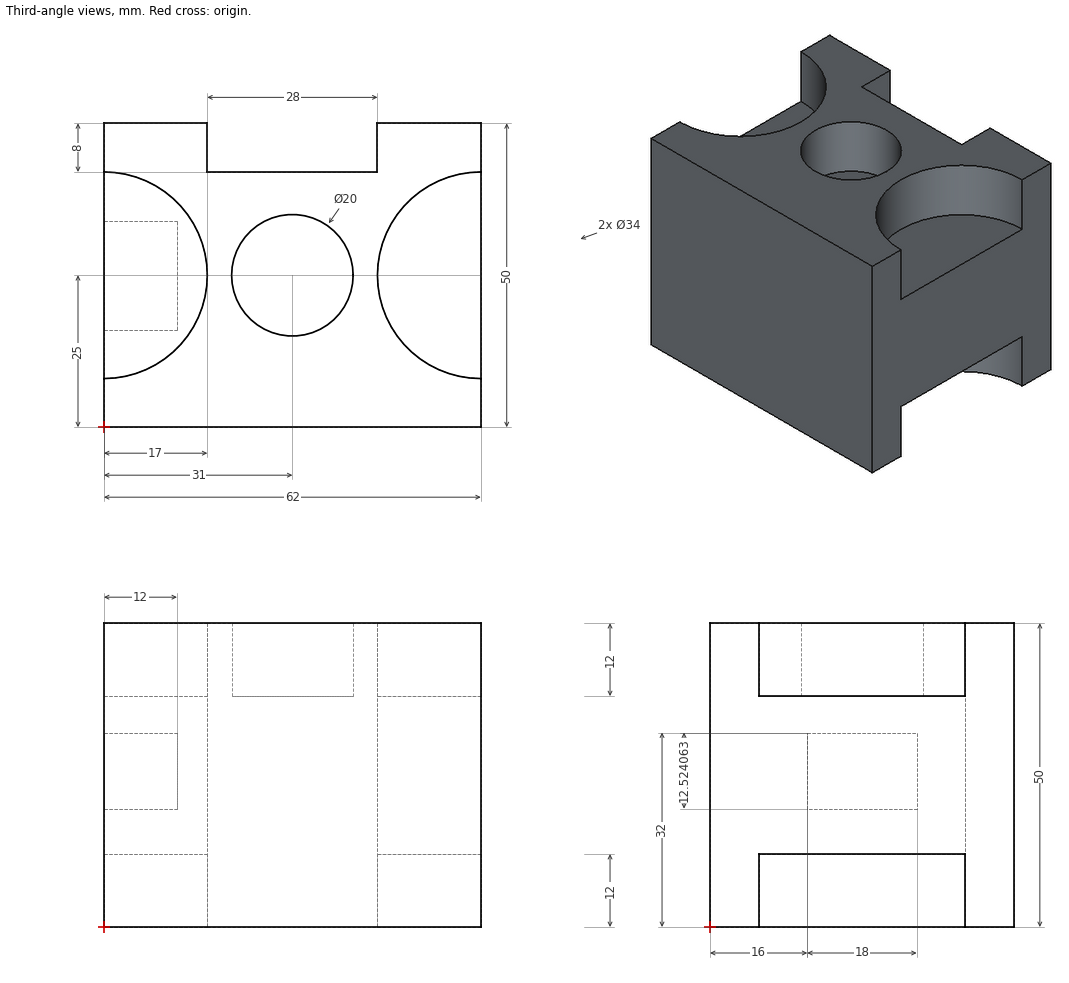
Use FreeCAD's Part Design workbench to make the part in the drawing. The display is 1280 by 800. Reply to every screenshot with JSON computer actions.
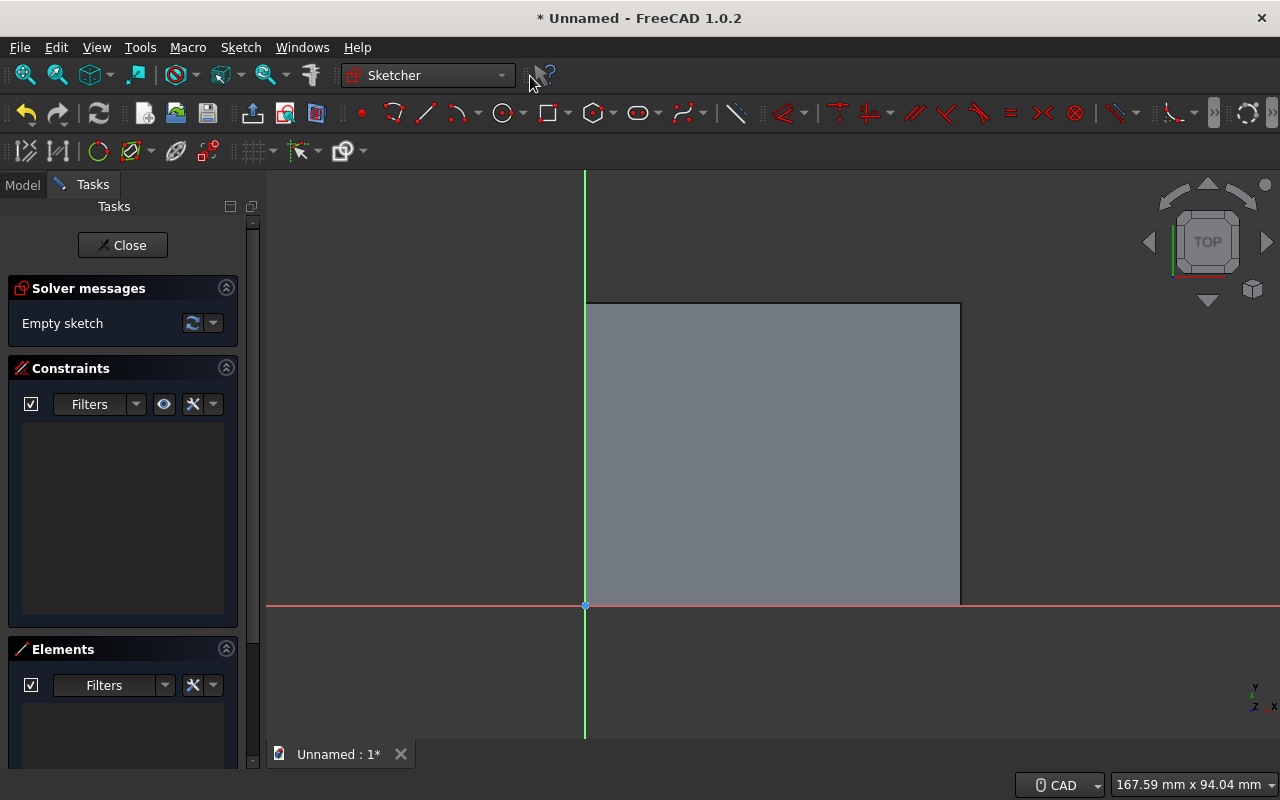
{"action": "left_click", "coordinate": [504, 114]}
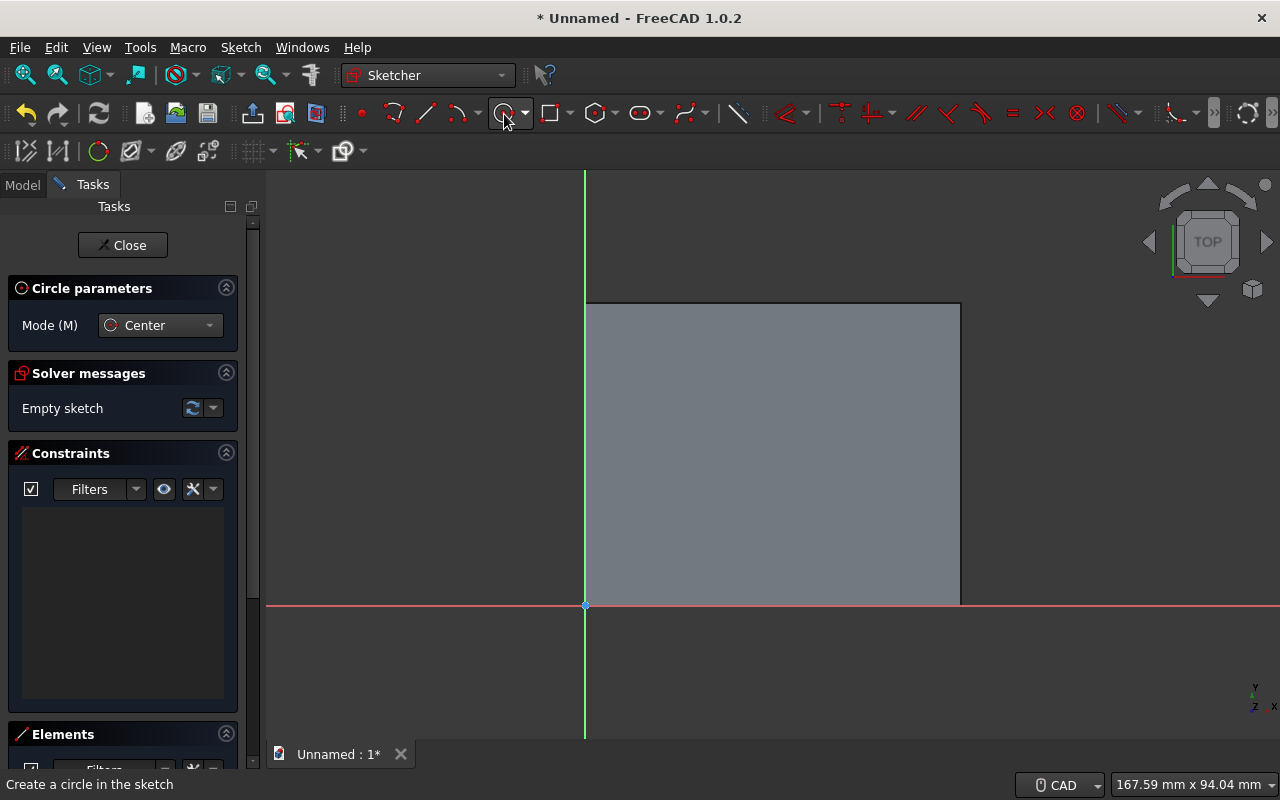
{"action": "left_click", "coordinate": [961, 455]}
{"action": "left_click", "coordinate": [1033, 382]}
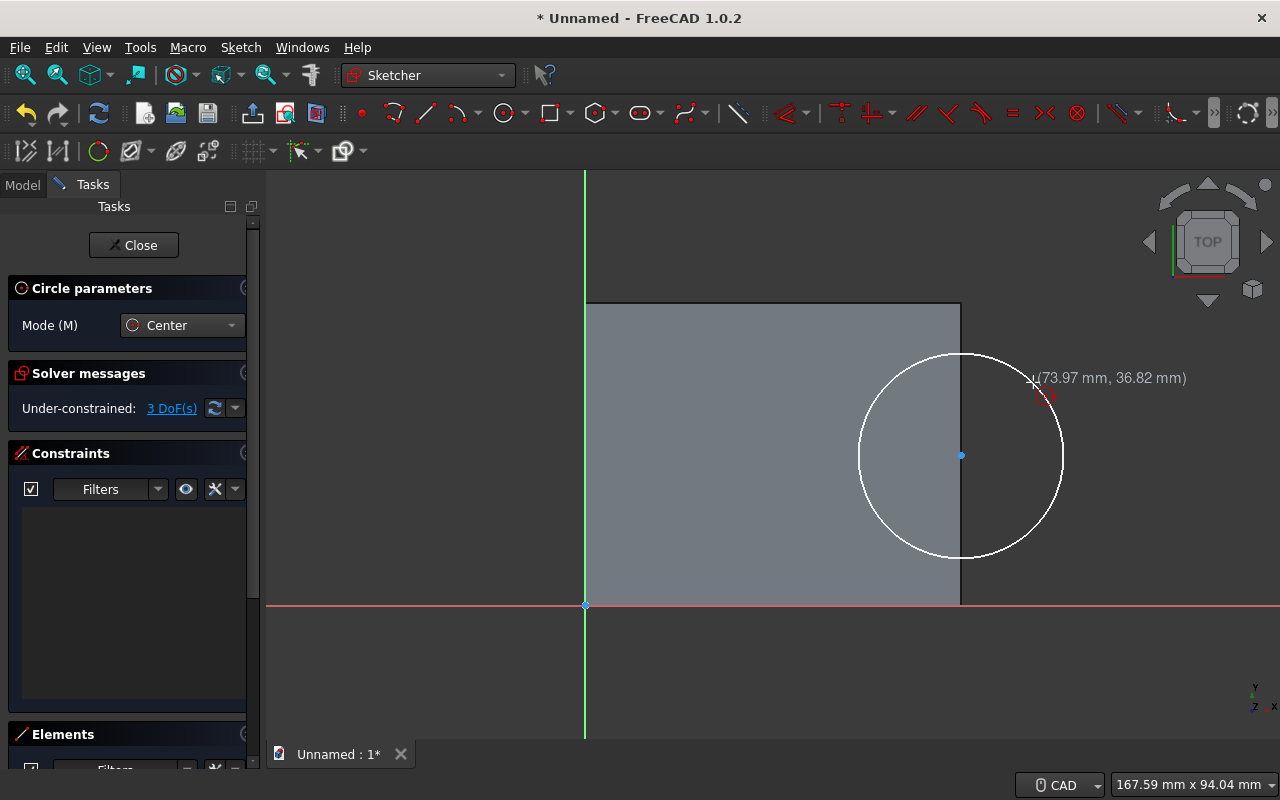
{"action": "left_click", "coordinate": [585, 455]}
{"action": "left_click", "coordinate": [658, 382]}
{"action": "key", "text": "Escape"}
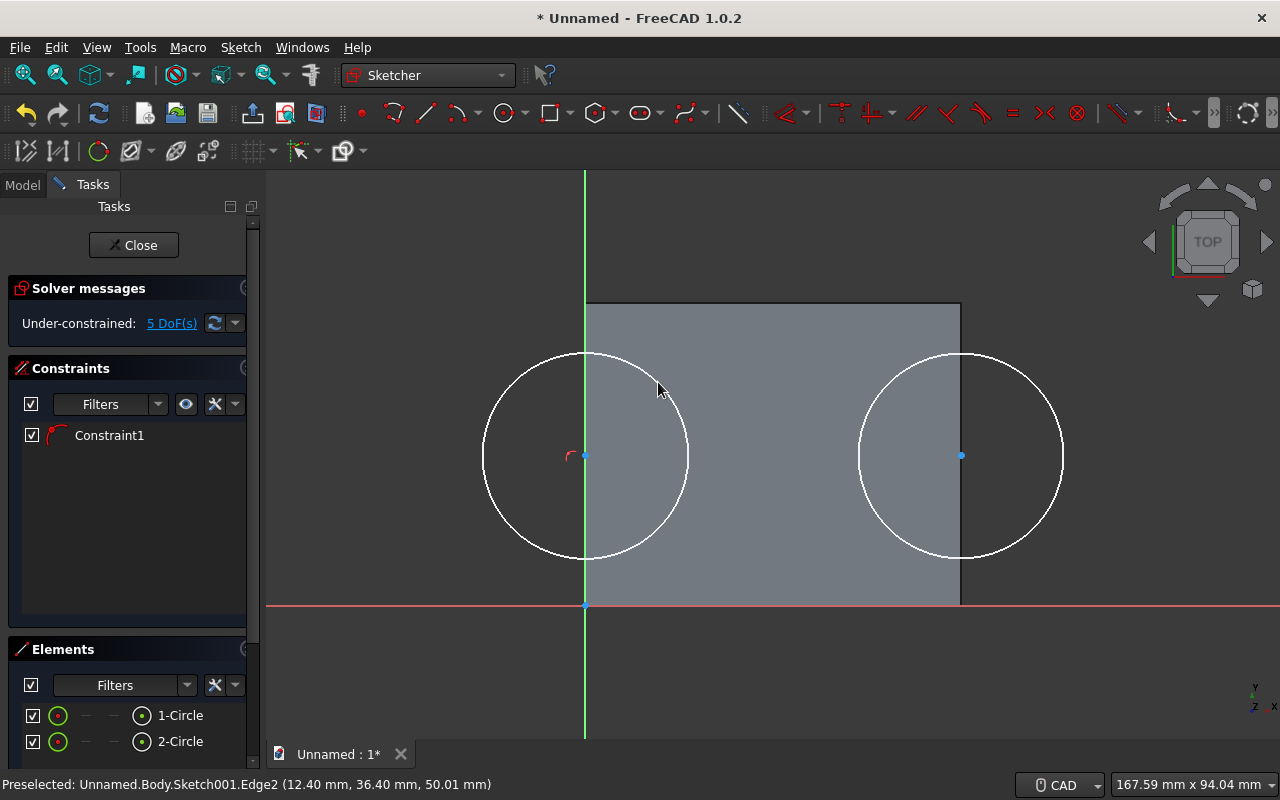
{"action": "left_click", "coordinate": [1033, 383]}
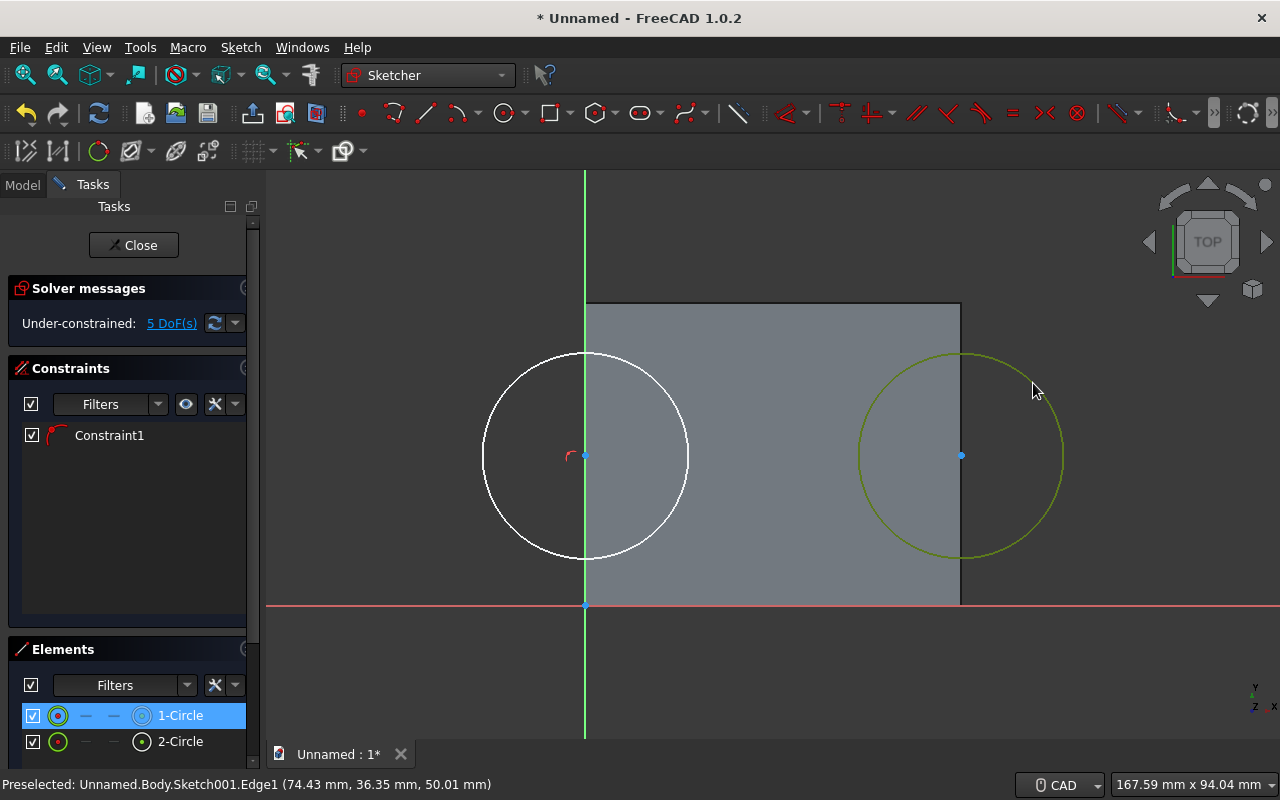
{"action": "left_click", "coordinate": [658, 383]}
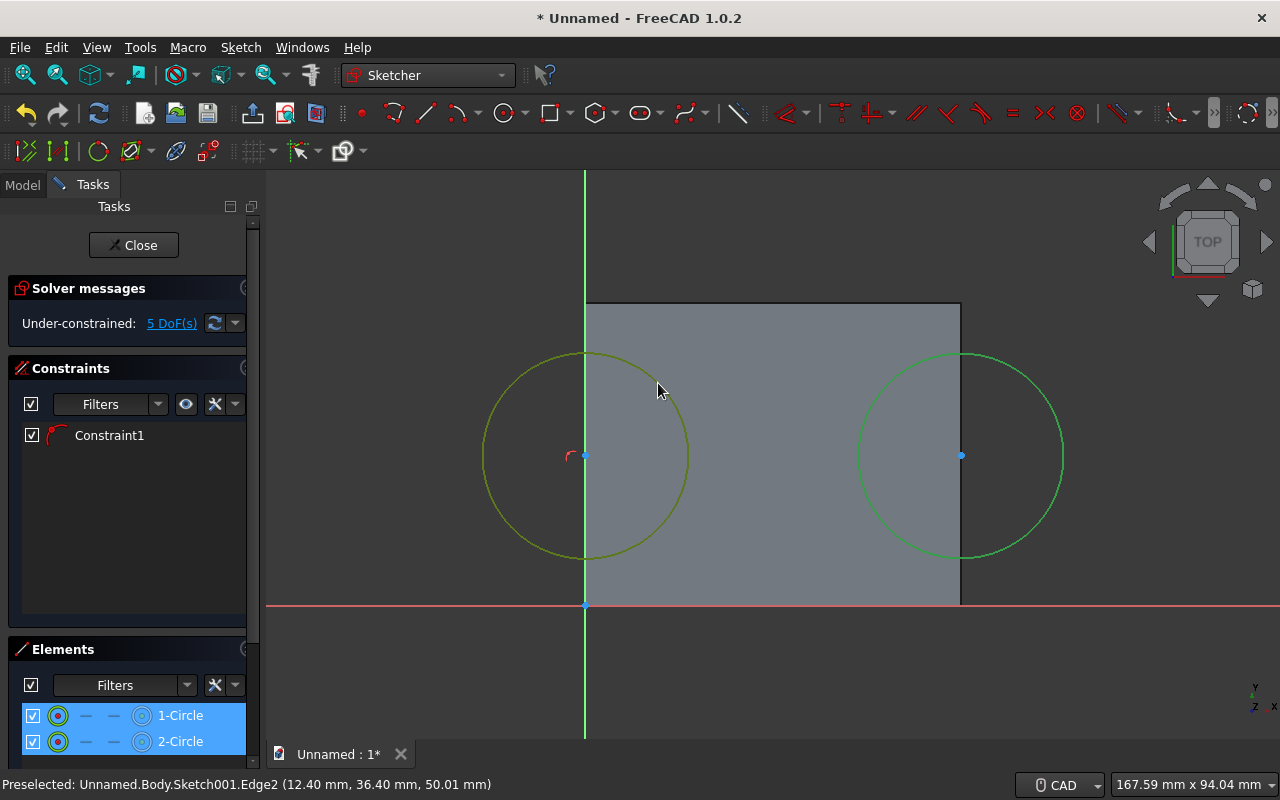
{"action": "left_click", "coordinate": [1014, 114]}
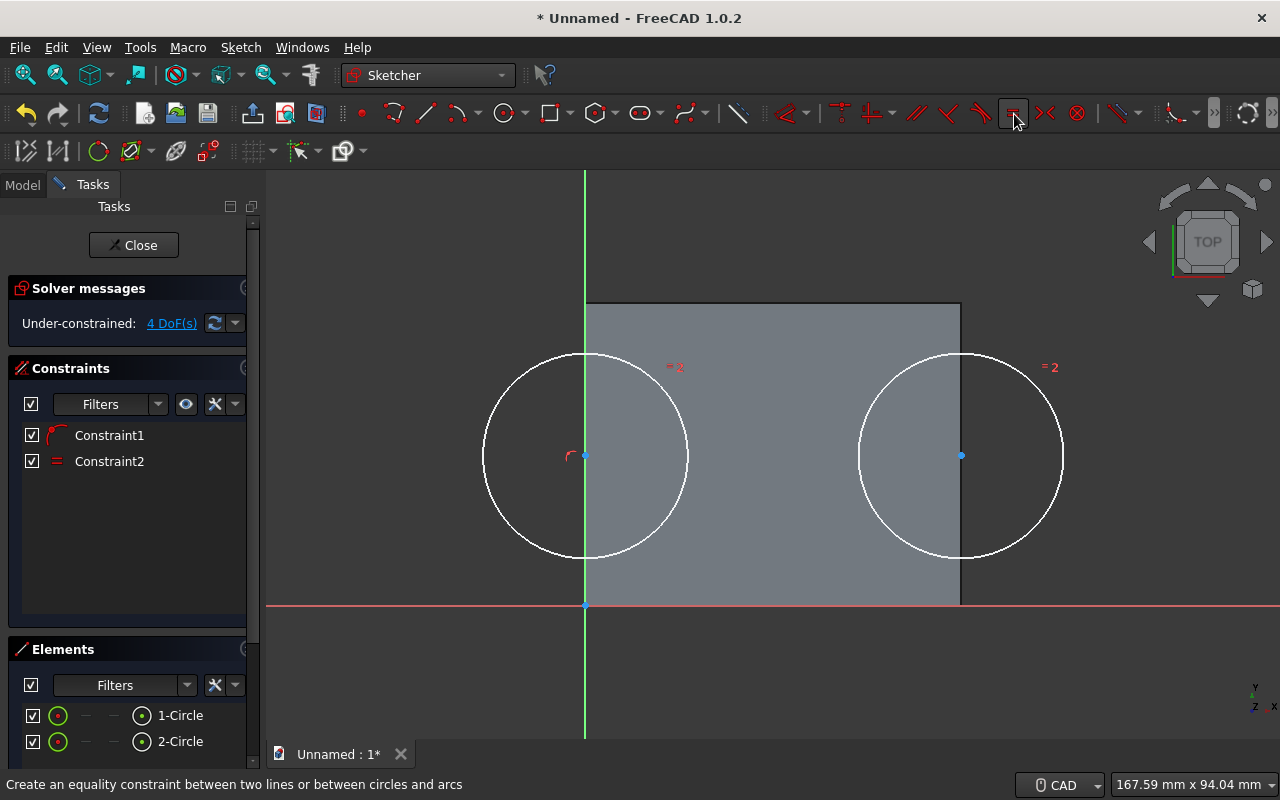
{"action": "left_click", "coordinate": [961, 456]}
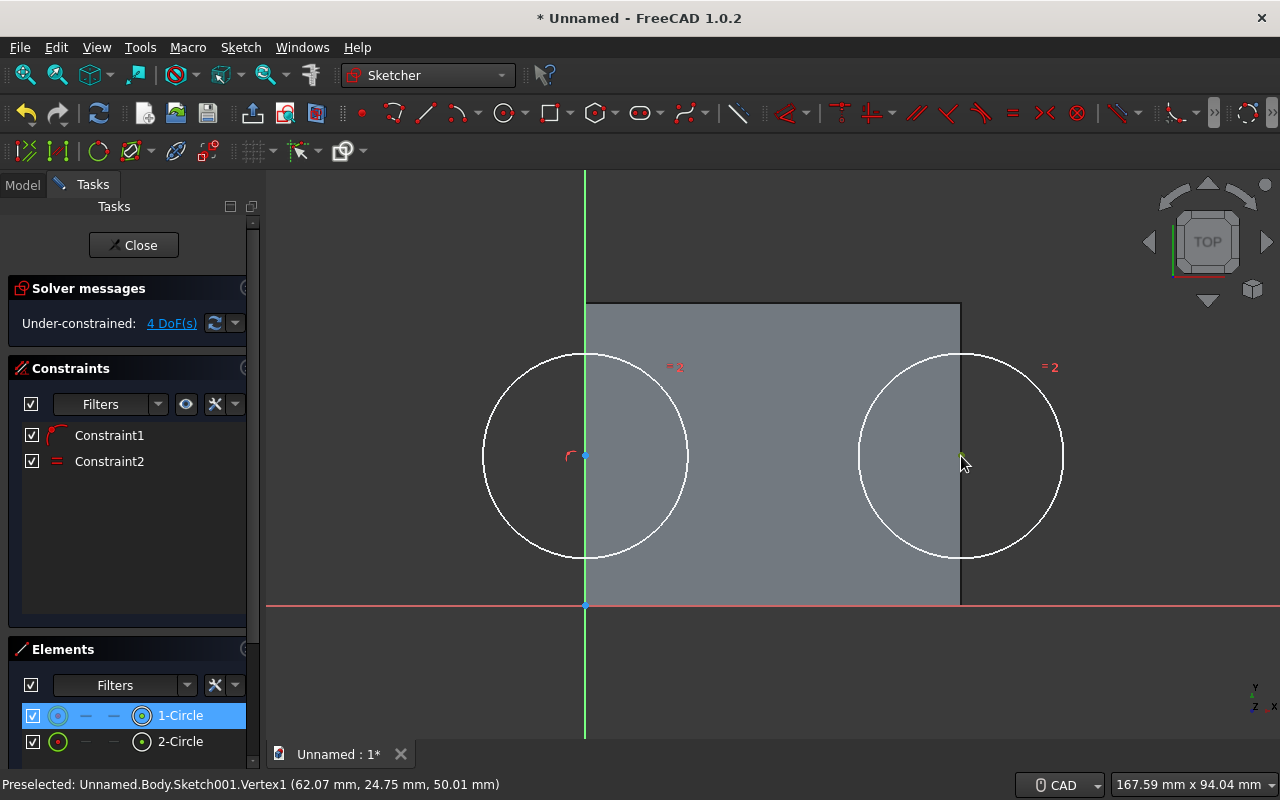
{"action": "left_click", "coordinate": [585, 456]}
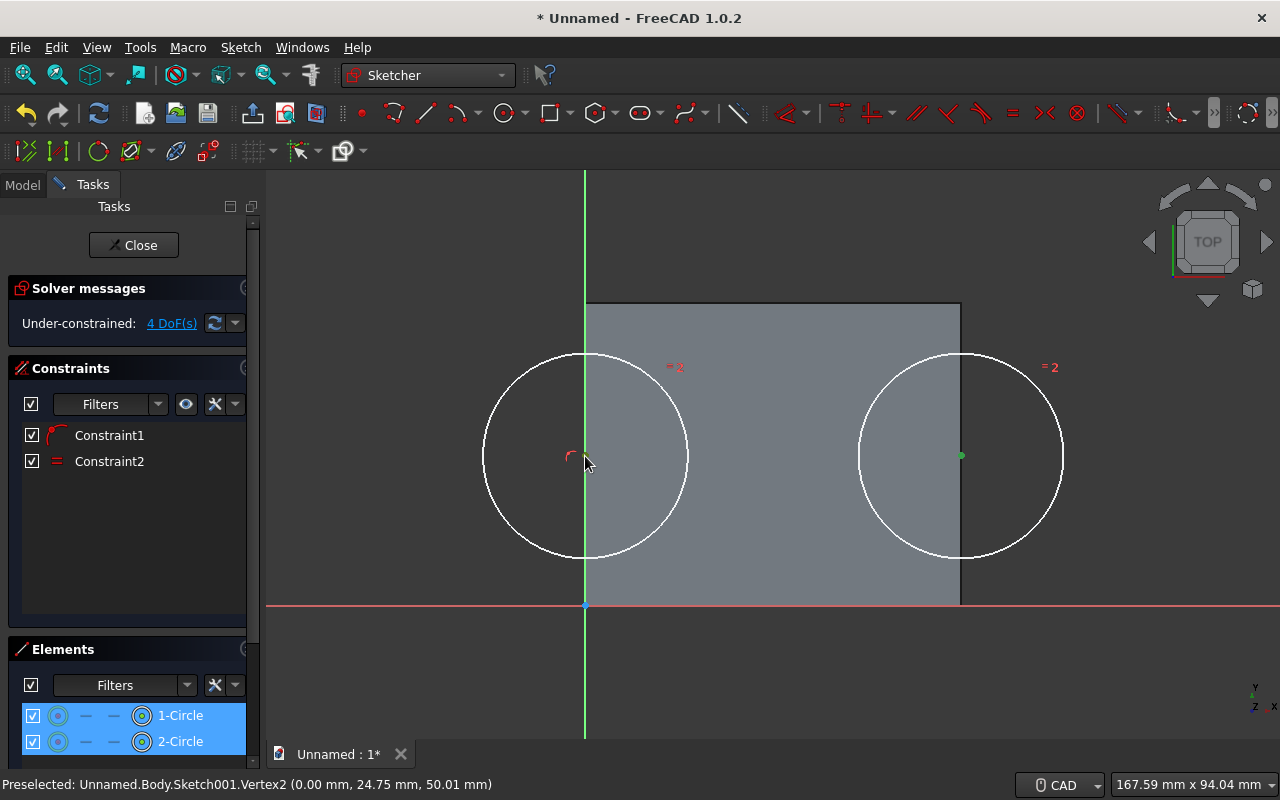
{"action": "key", "text": "h"}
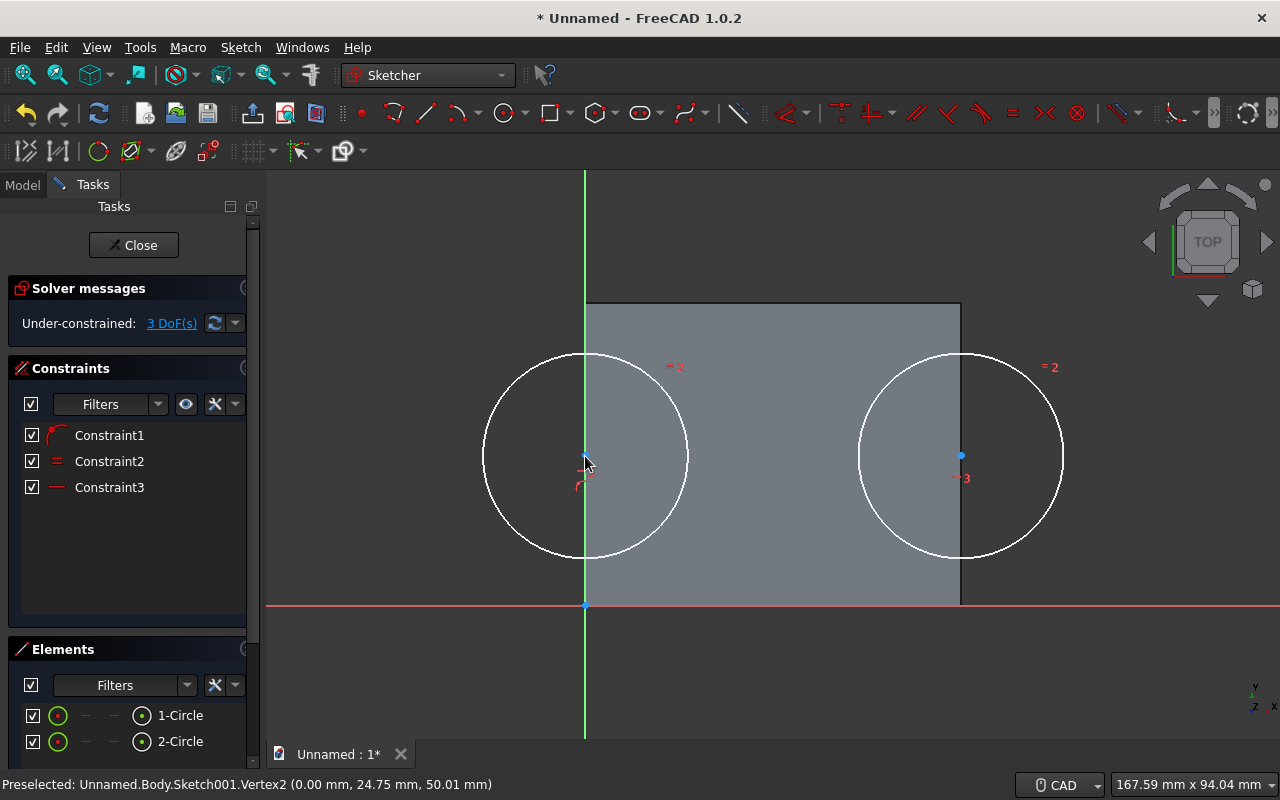
{"action": "left_click", "coordinate": [786, 114]}